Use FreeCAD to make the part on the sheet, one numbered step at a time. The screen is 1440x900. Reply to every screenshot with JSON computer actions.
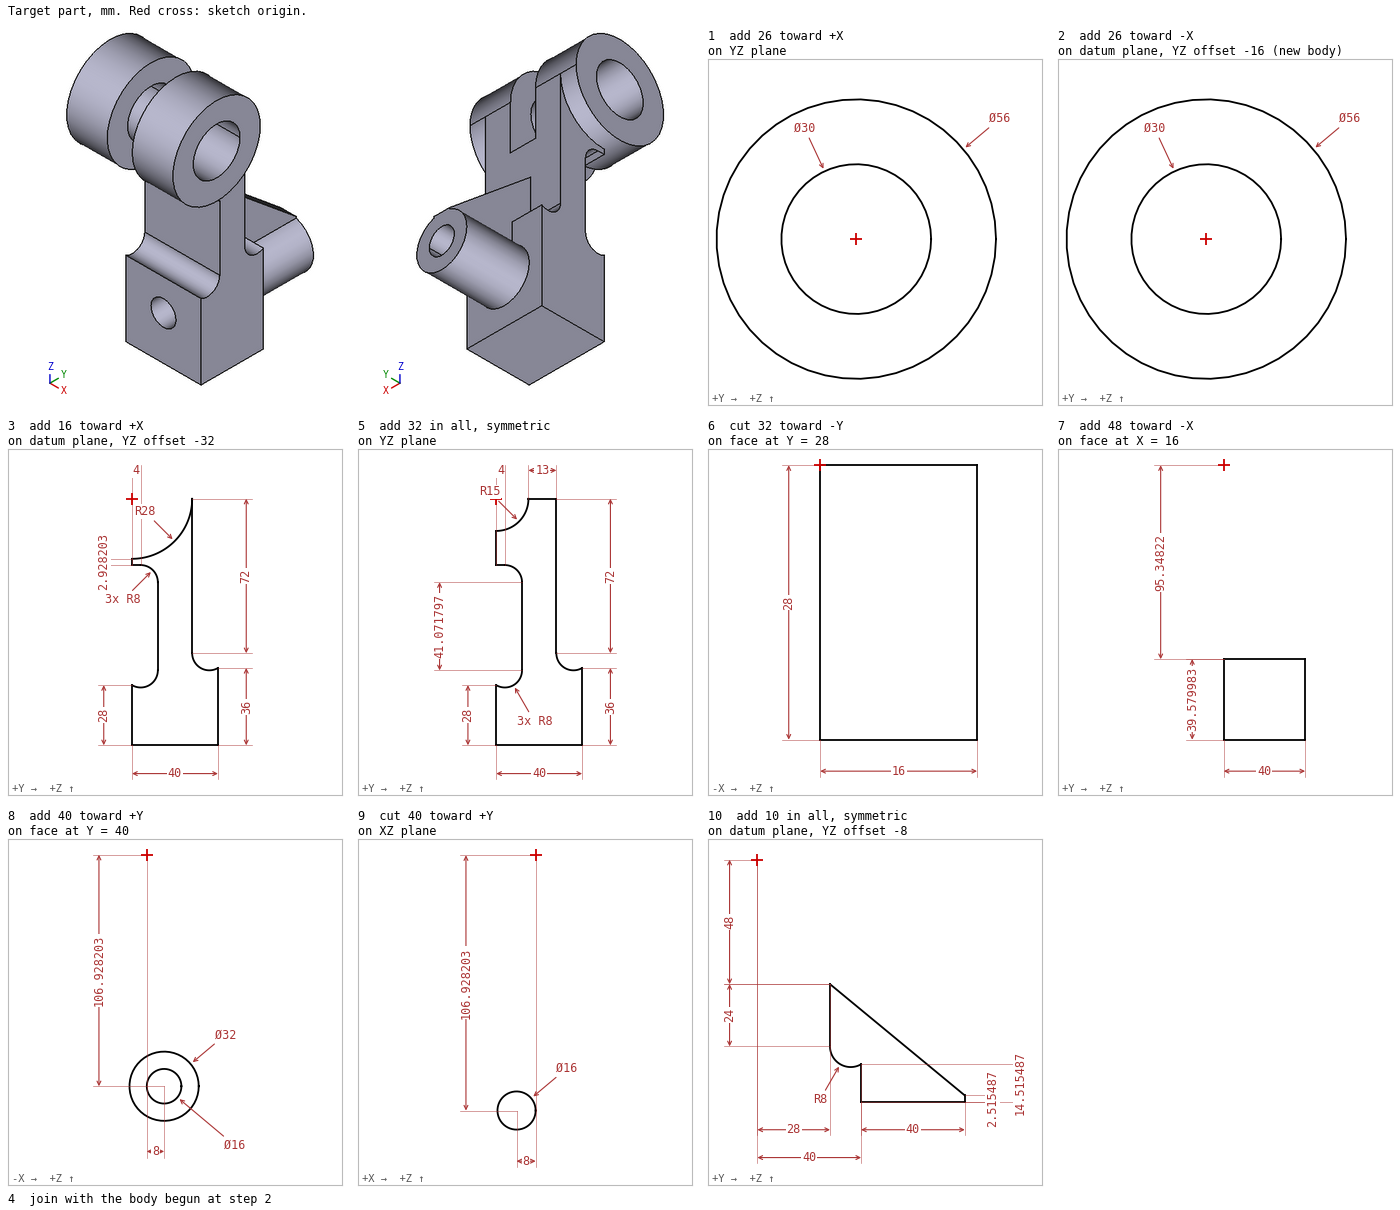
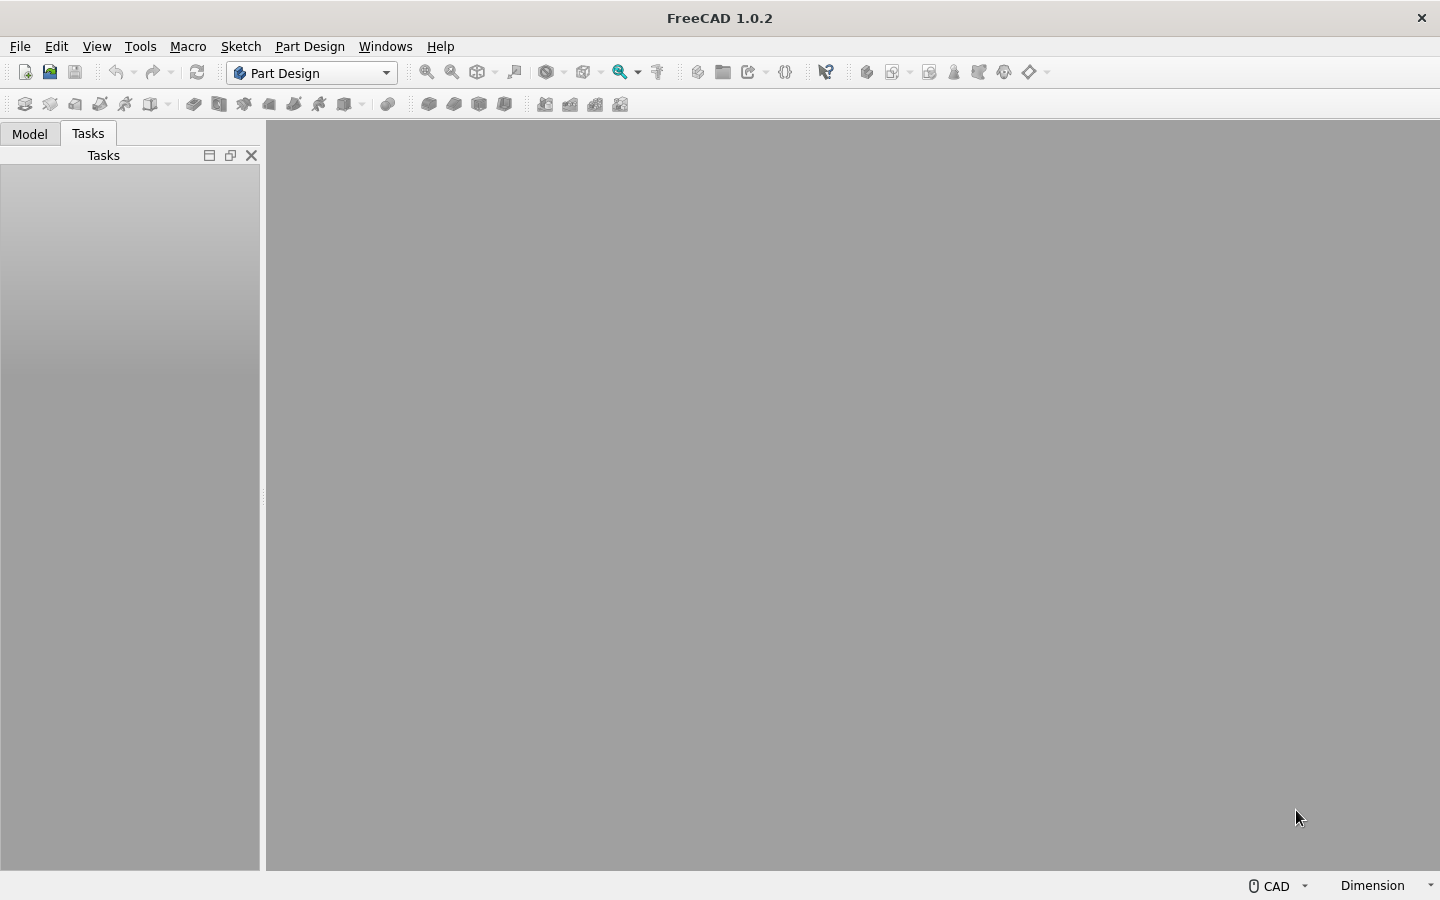
{"action": "key", "text": "ctrl+n"}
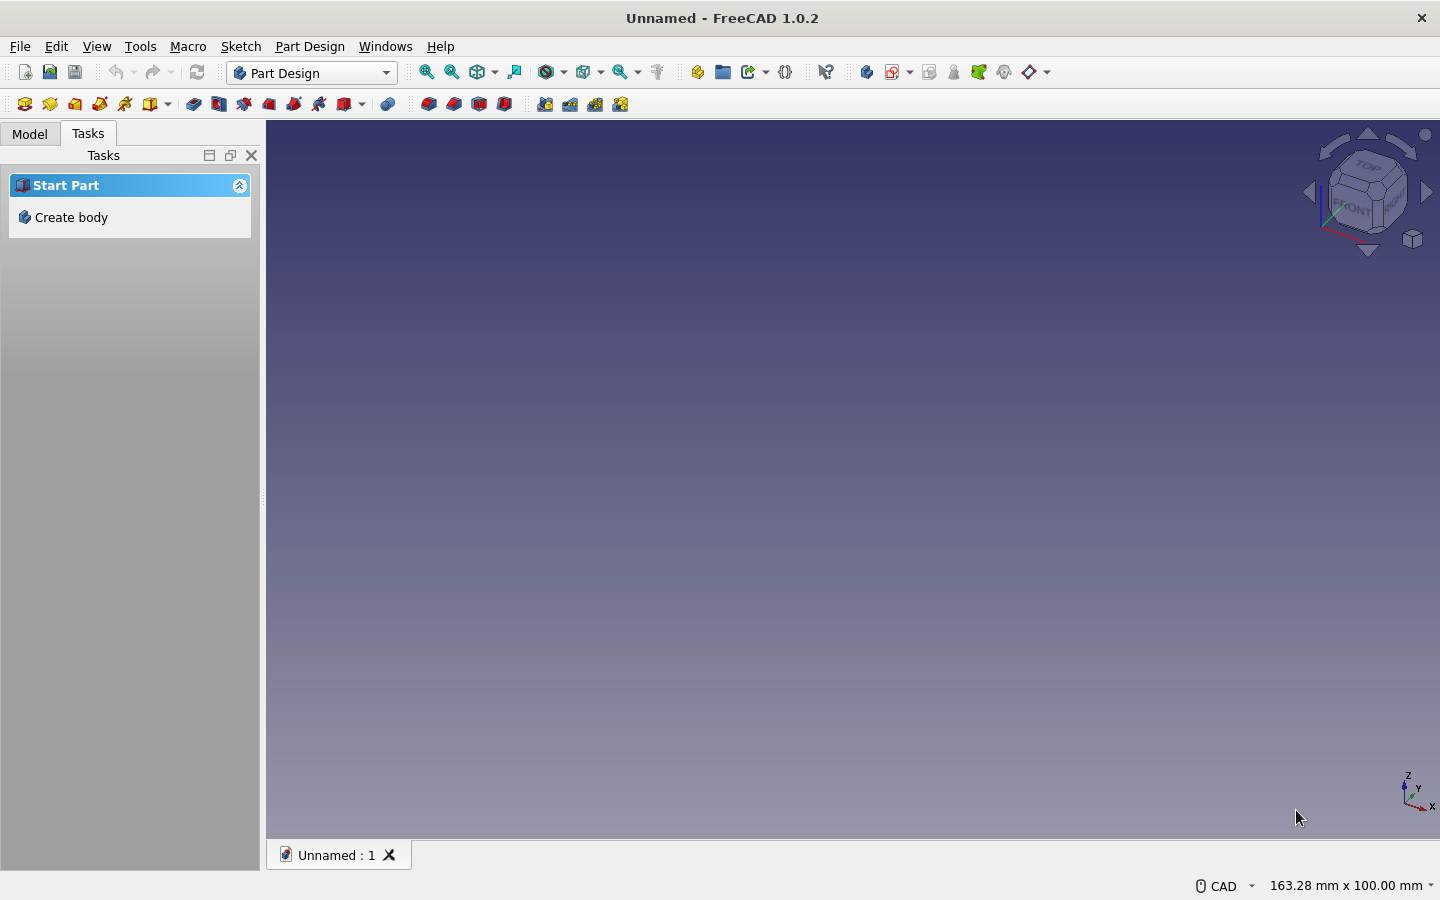
{"action": "left_click", "coordinate": [892, 72]}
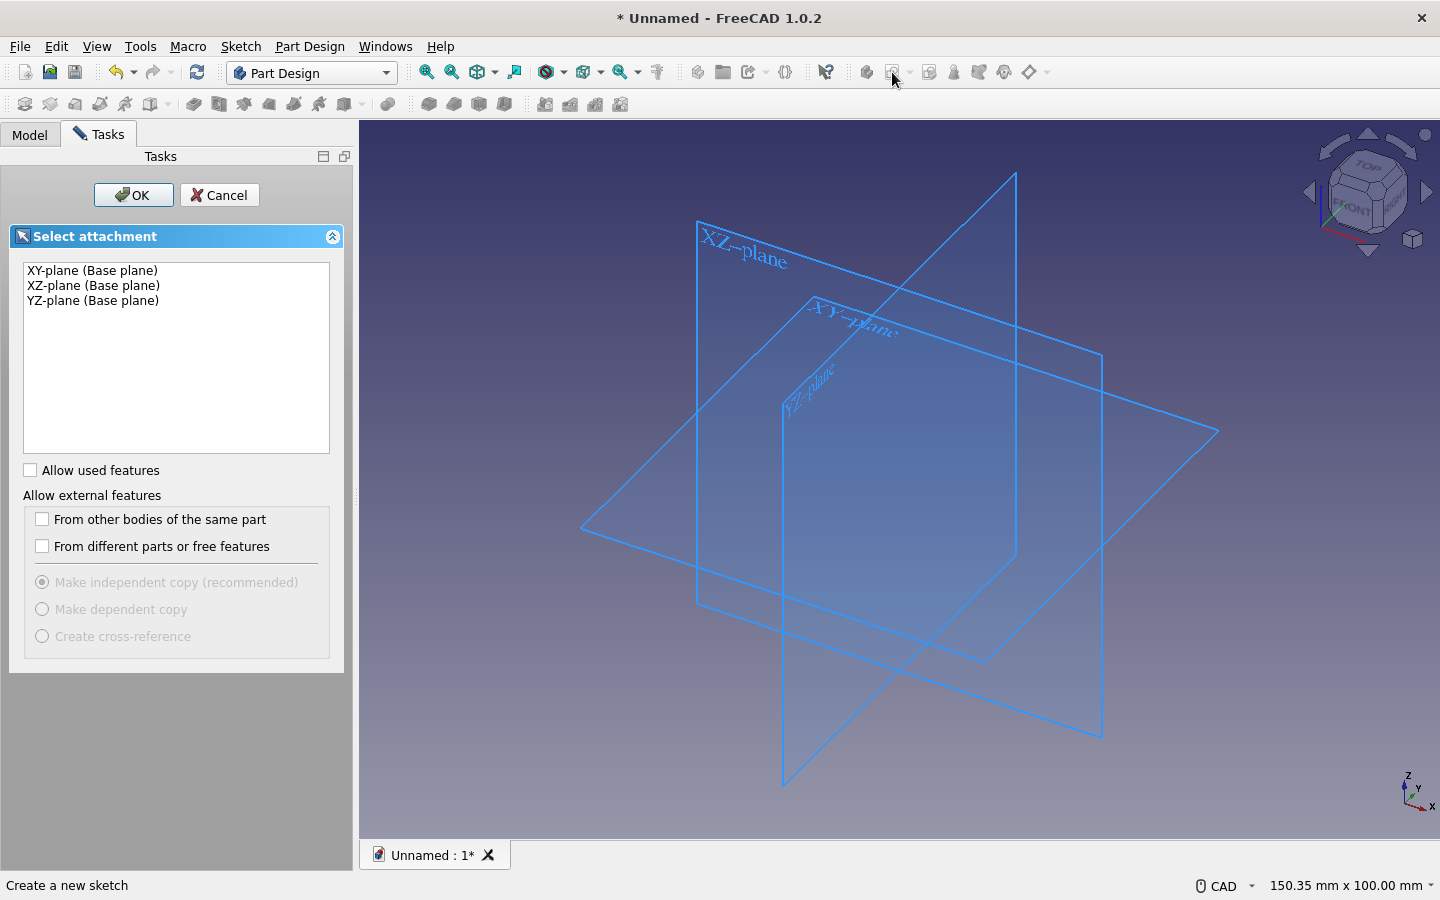
{"action": "left_click", "coordinate": [84, 300]}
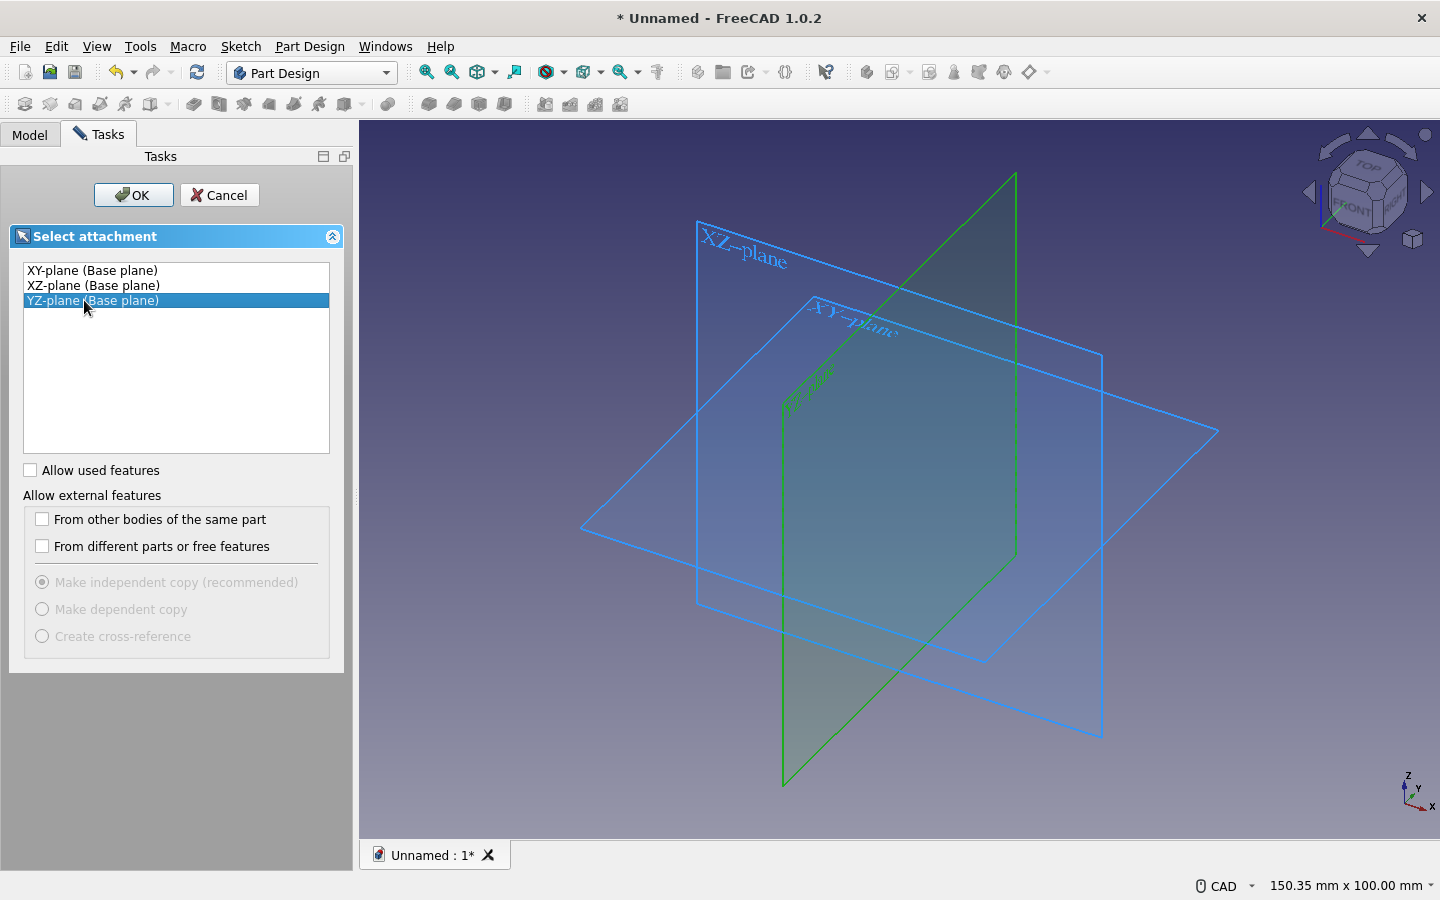
{"action": "left_click", "coordinate": [134, 195]}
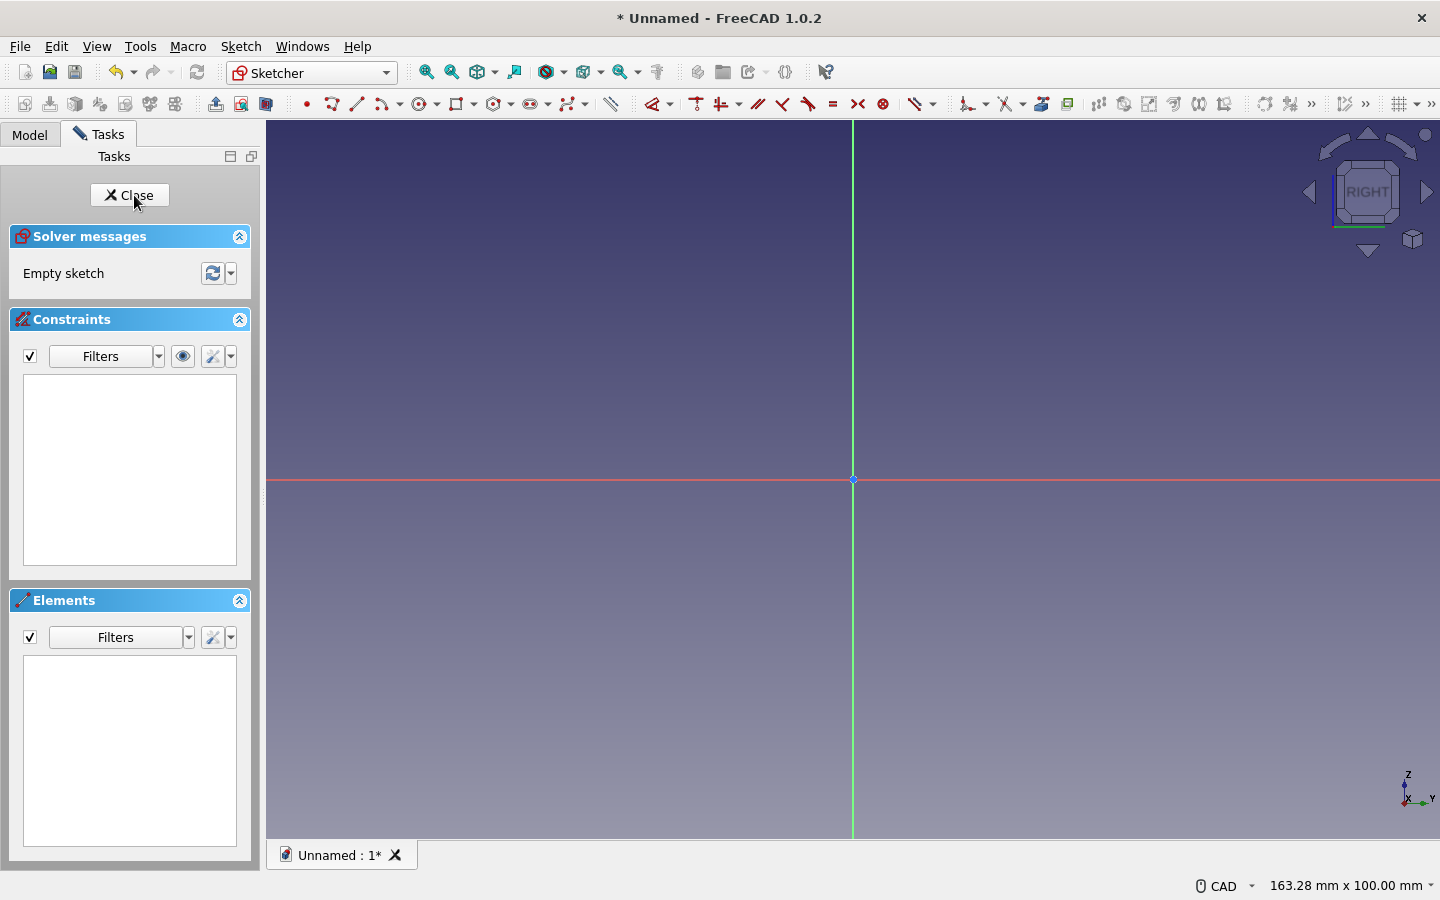
{"action": "left_click", "coordinate": [418, 104]}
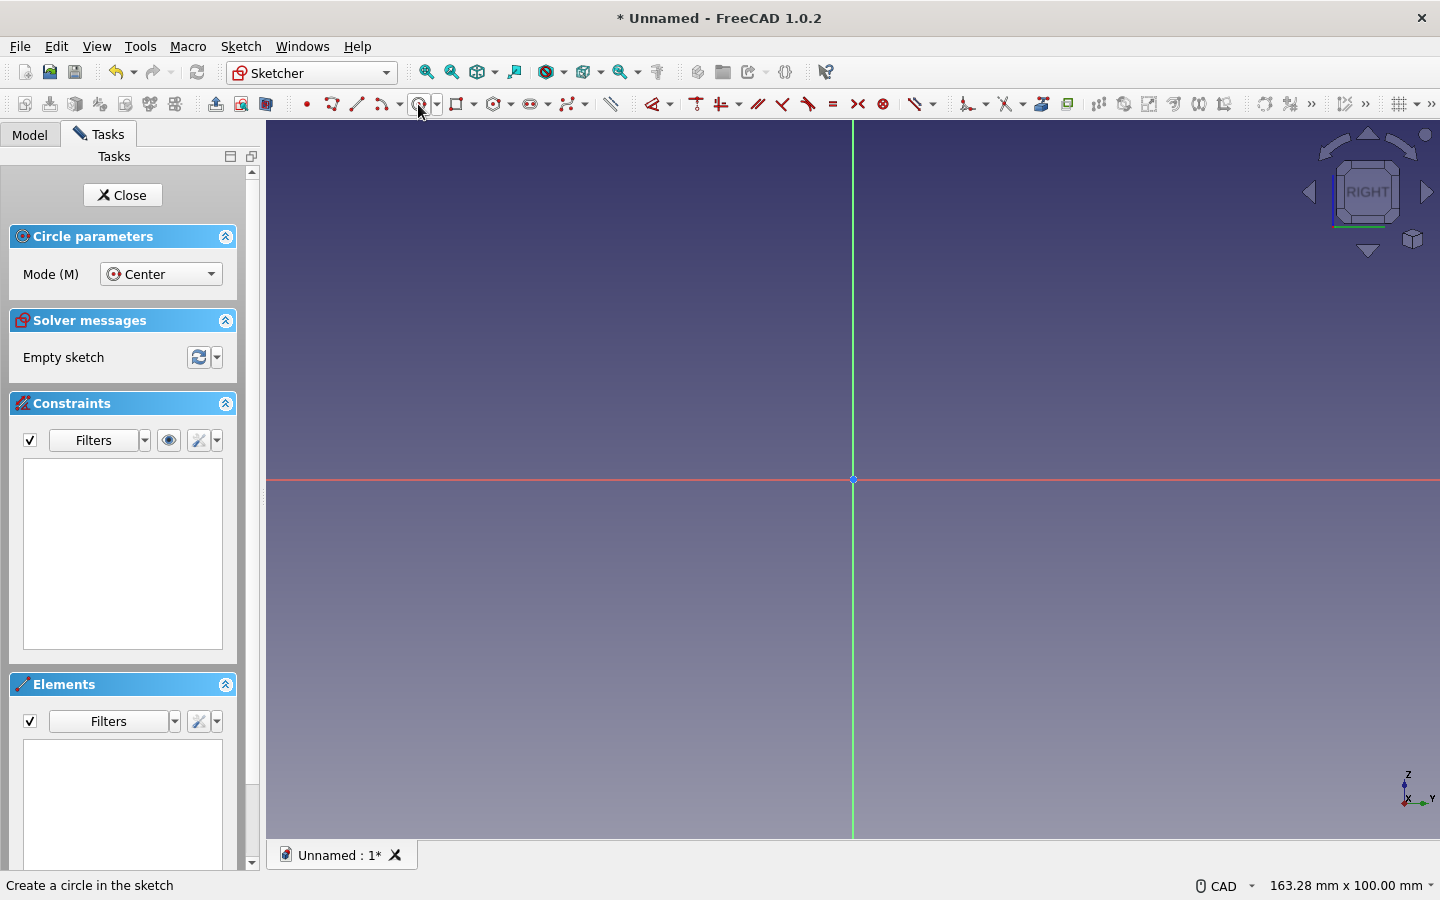
{"action": "left_click", "coordinate": [853, 480]}
{"action": "left_click", "coordinate": [995, 337]}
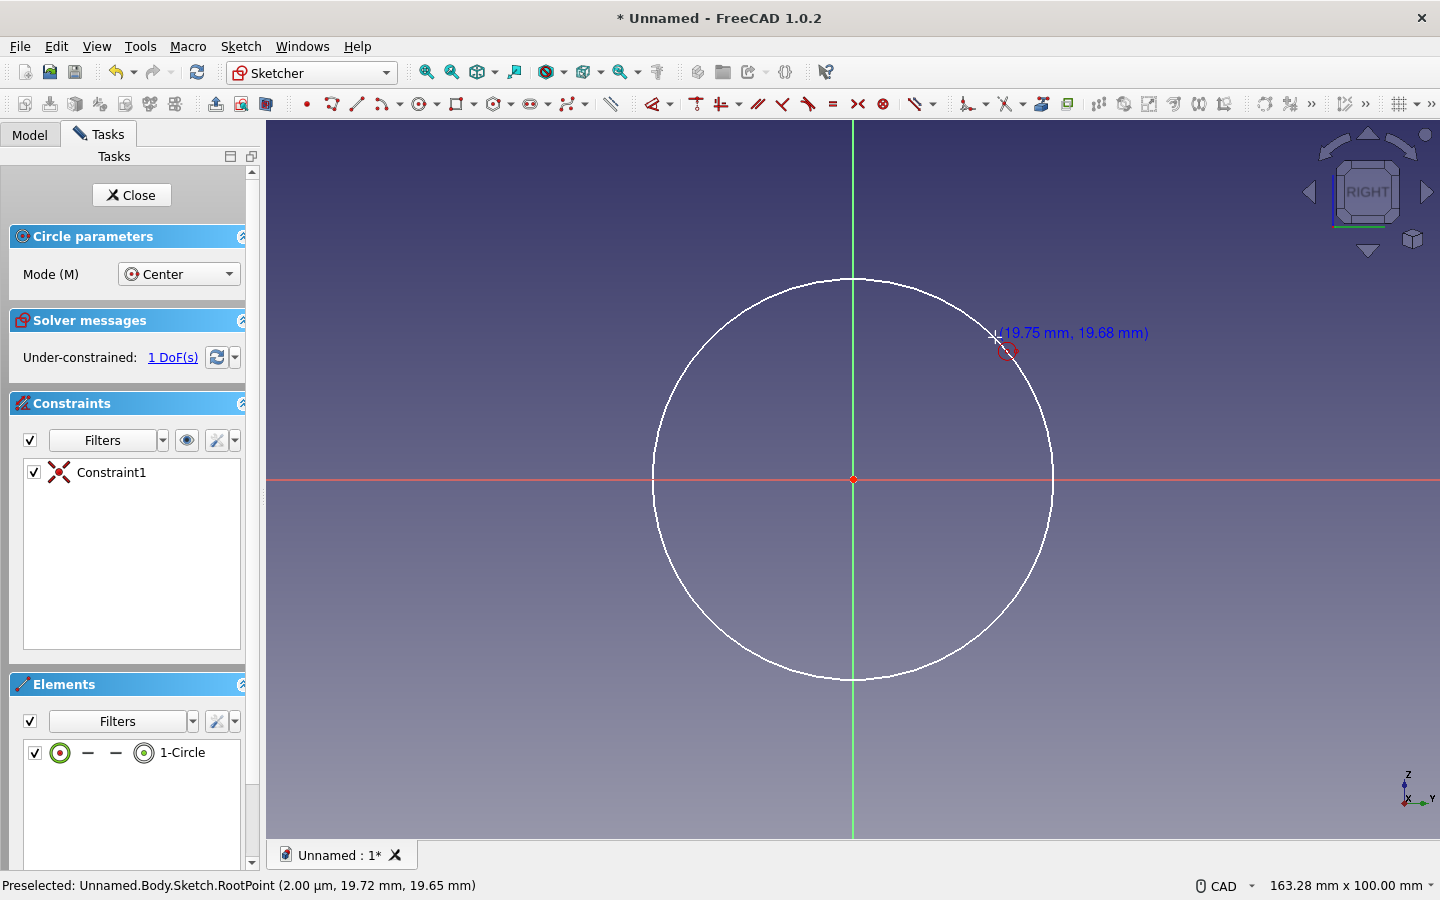
{"action": "left_click", "coordinate": [853, 480]}
{"action": "left_click", "coordinate": [929, 403]}
{"action": "key", "text": "Escape"}